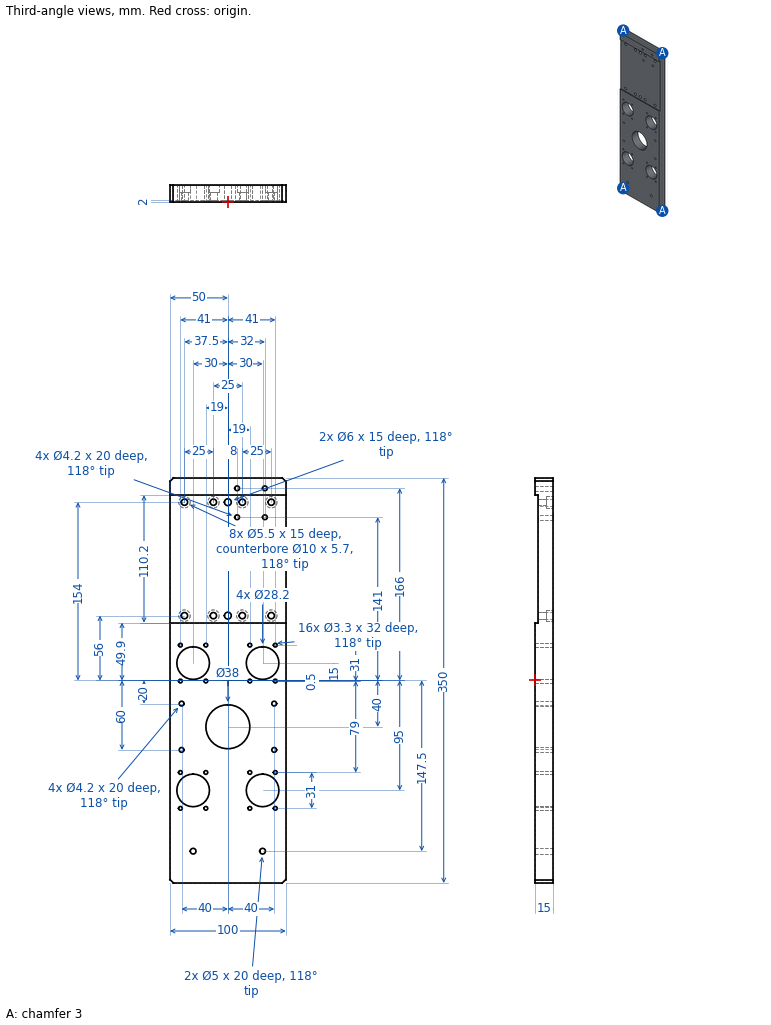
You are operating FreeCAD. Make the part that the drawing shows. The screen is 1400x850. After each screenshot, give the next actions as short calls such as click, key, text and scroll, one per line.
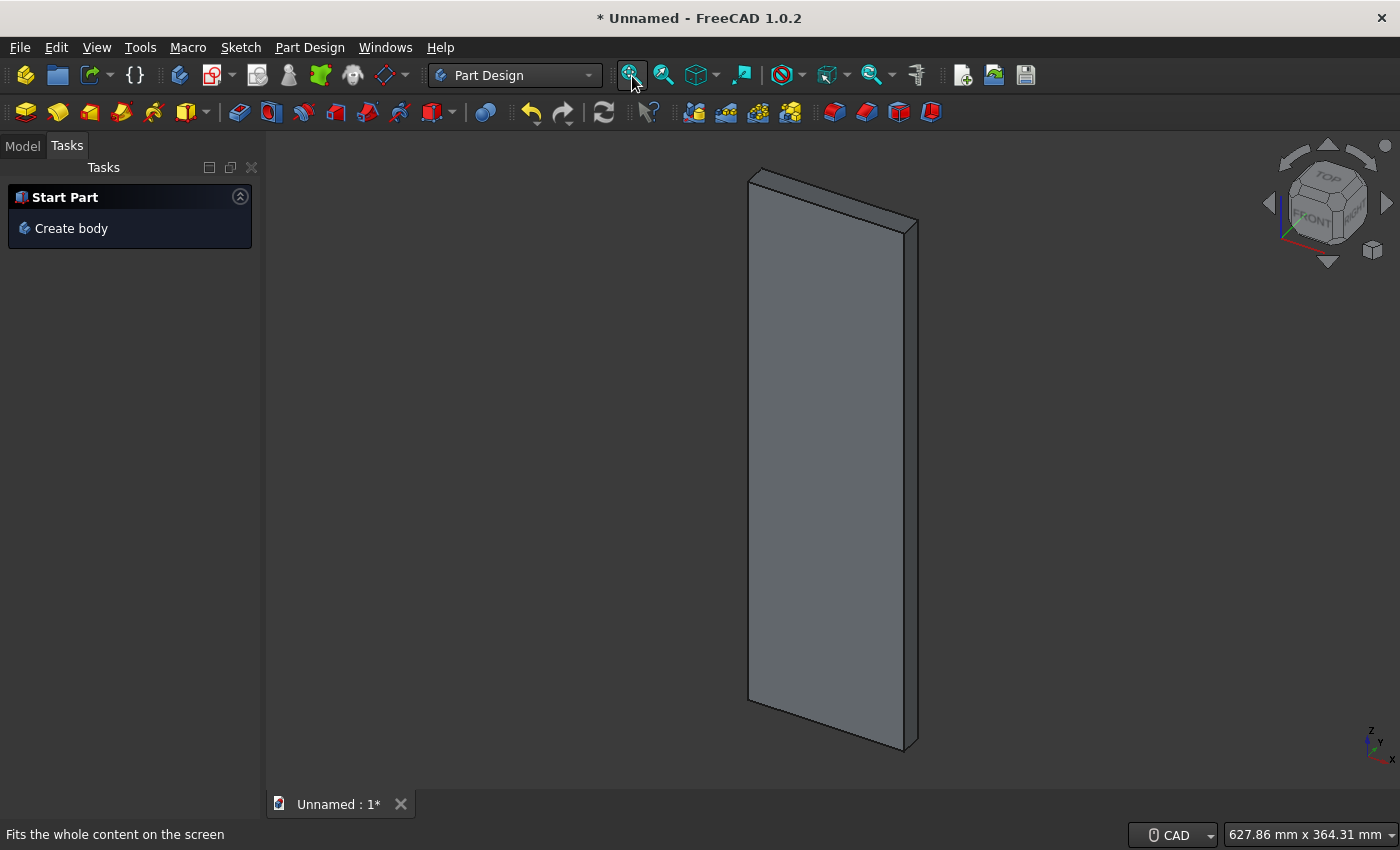
click(826, 318)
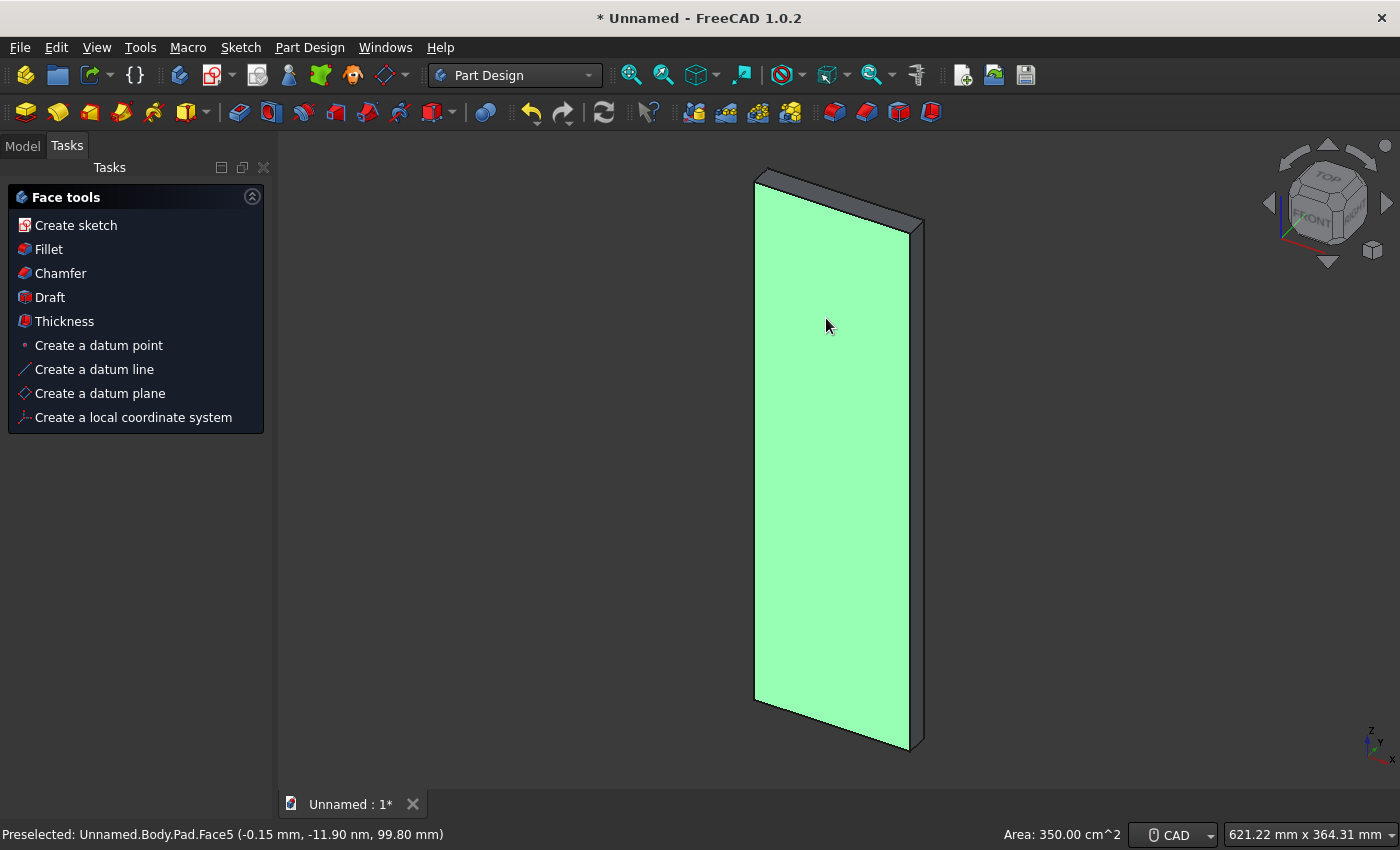
click(212, 76)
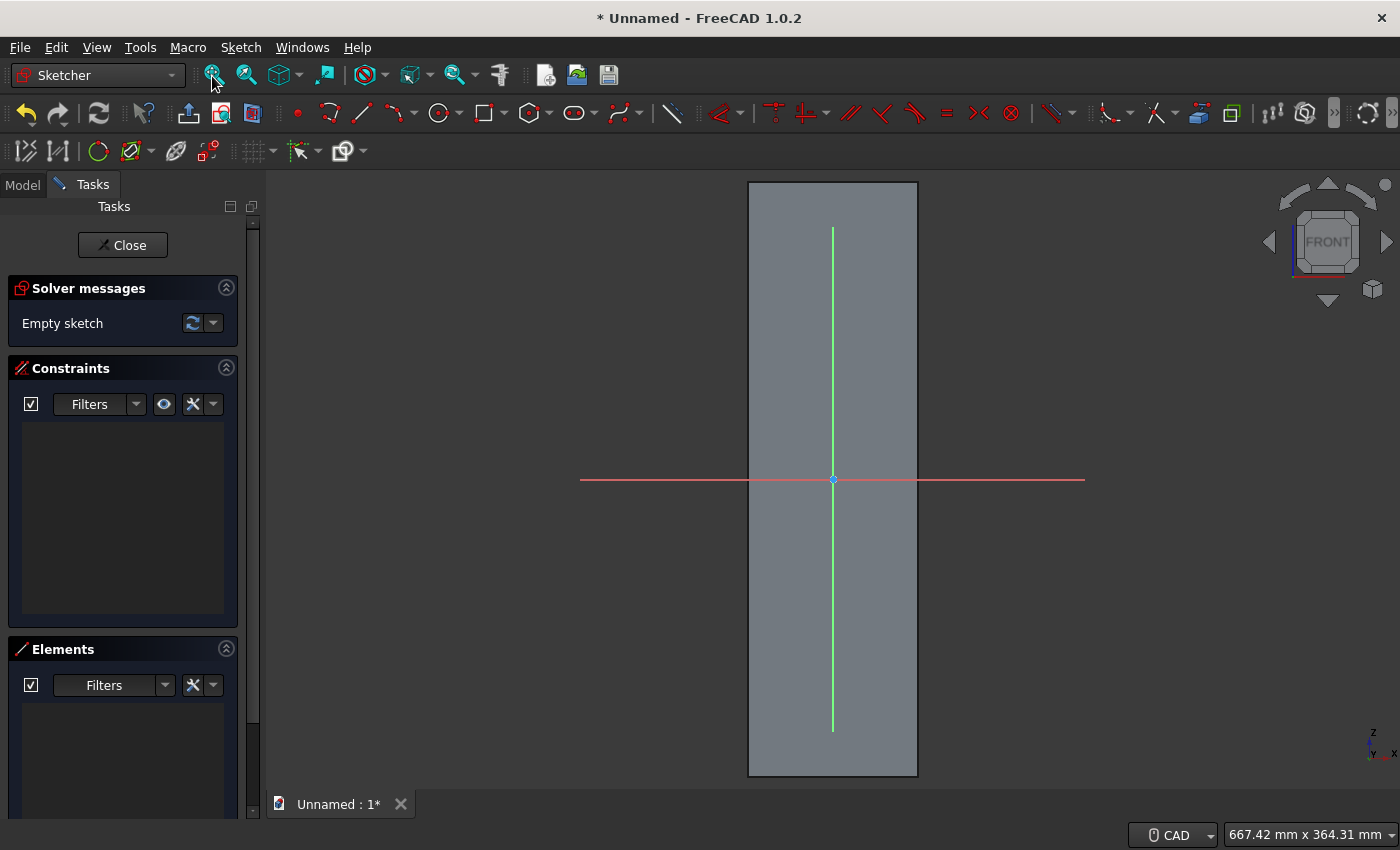
scroll(455, 761, down, 1)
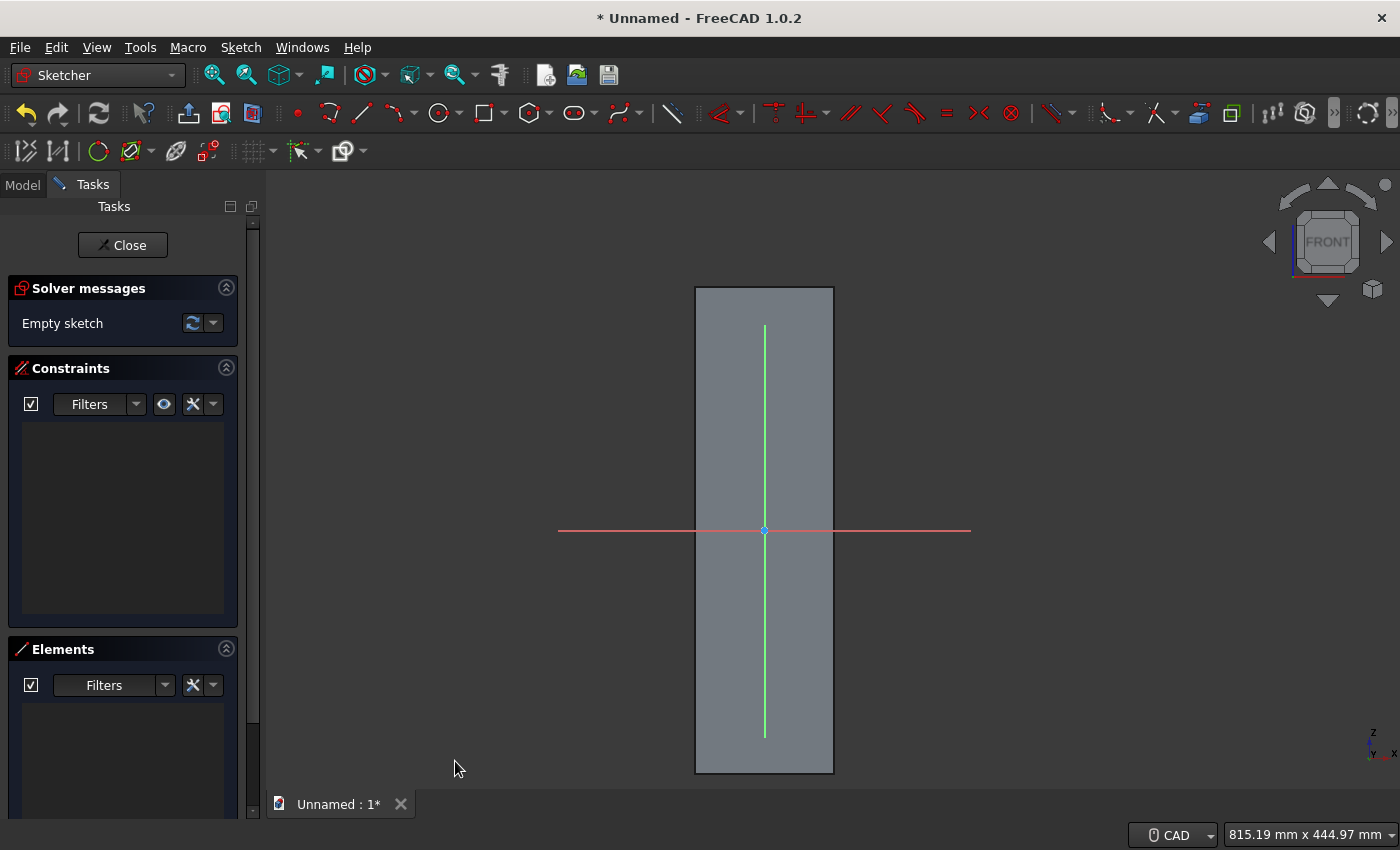
scroll(765, 346, up, 3)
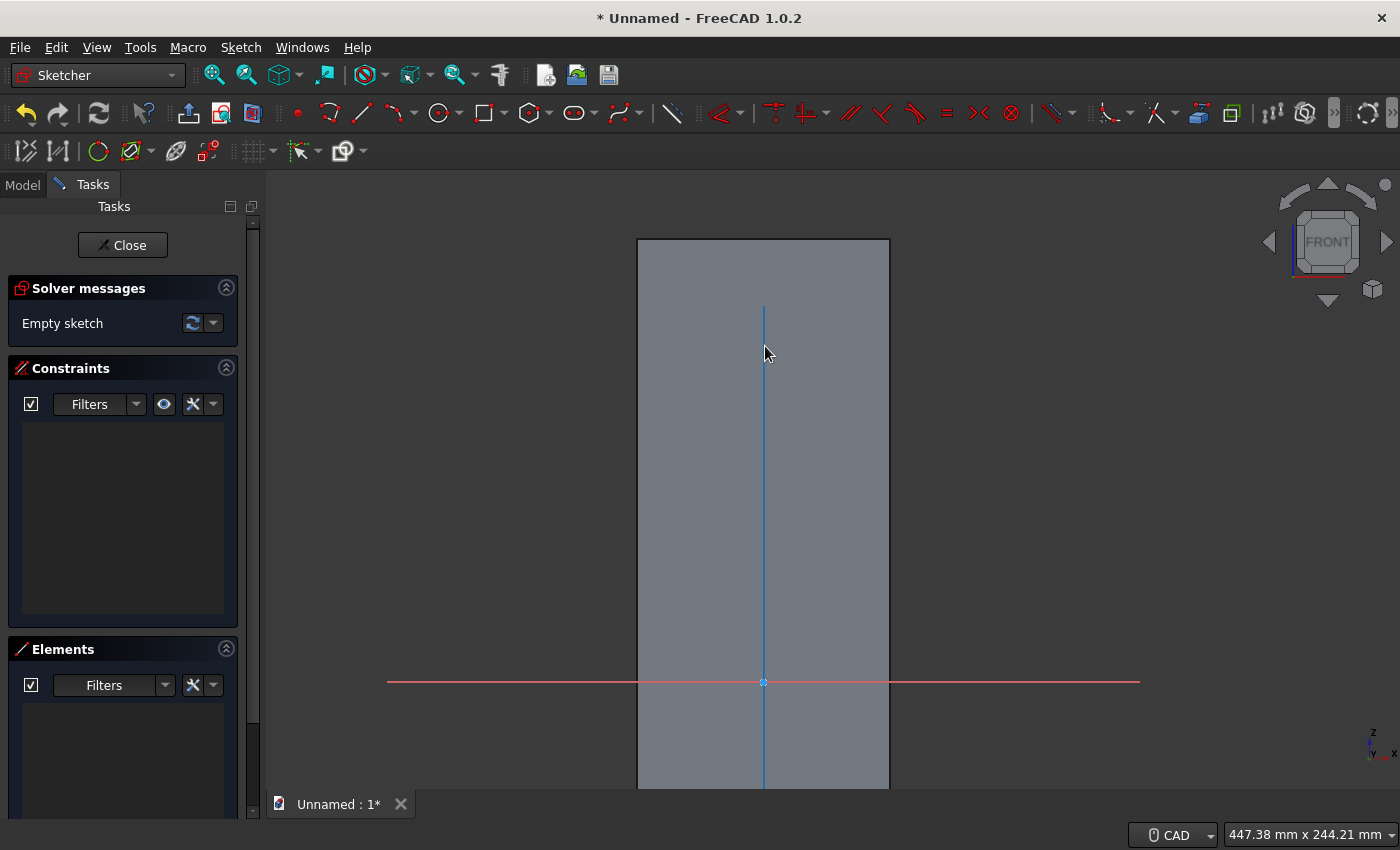
key(g)
key(r)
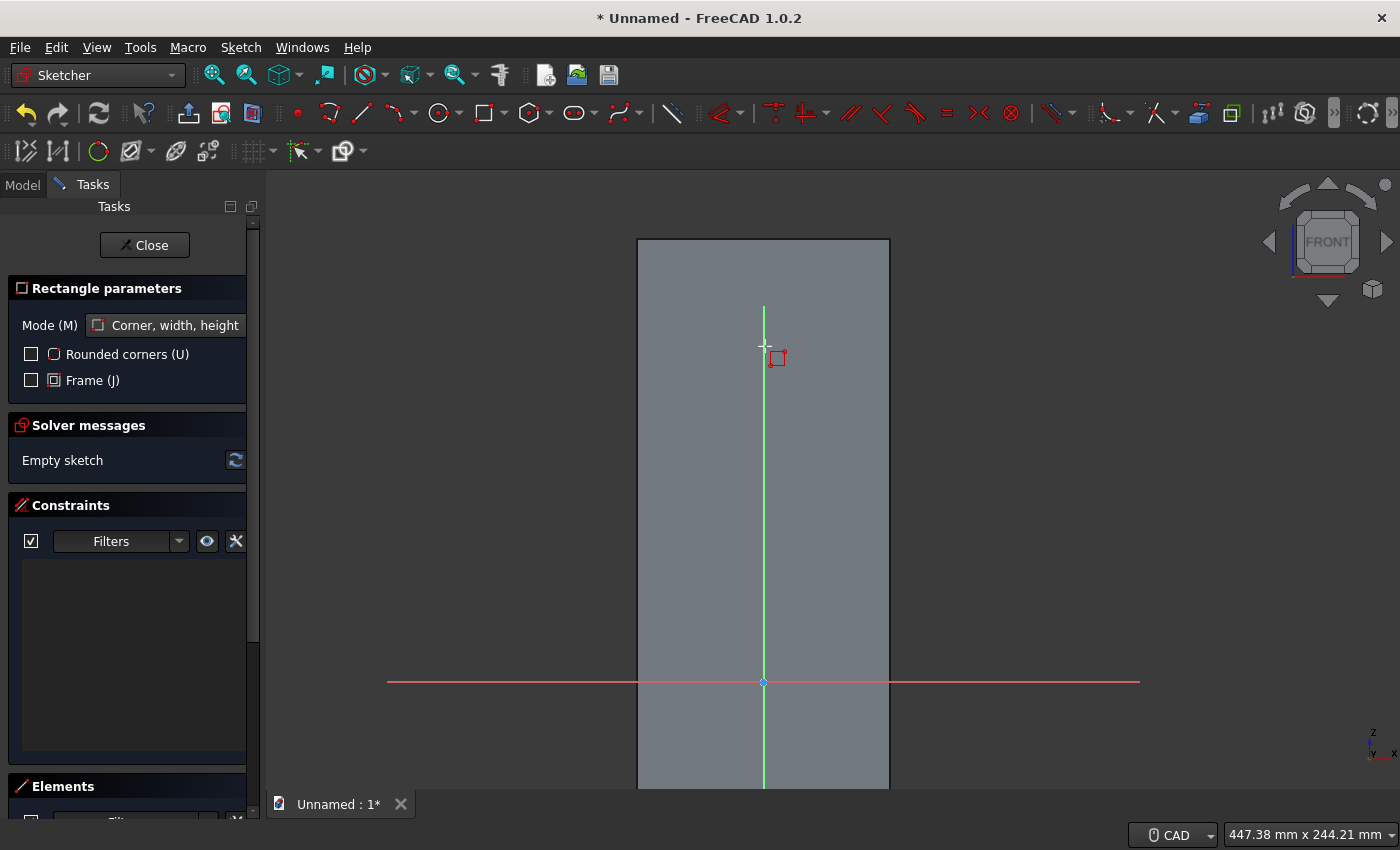
click(637, 277)
click(890, 556)
key(Escape)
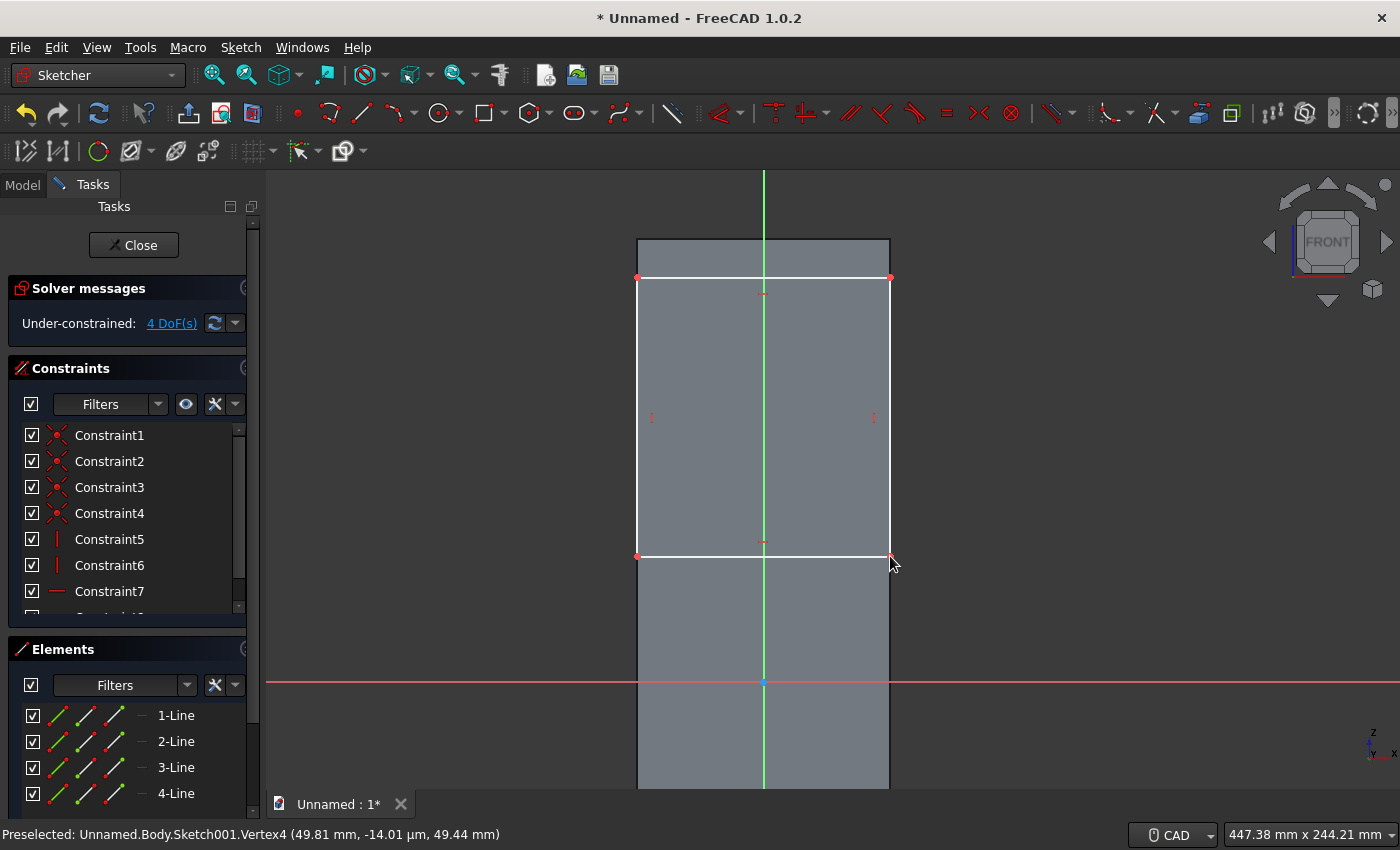
key(d)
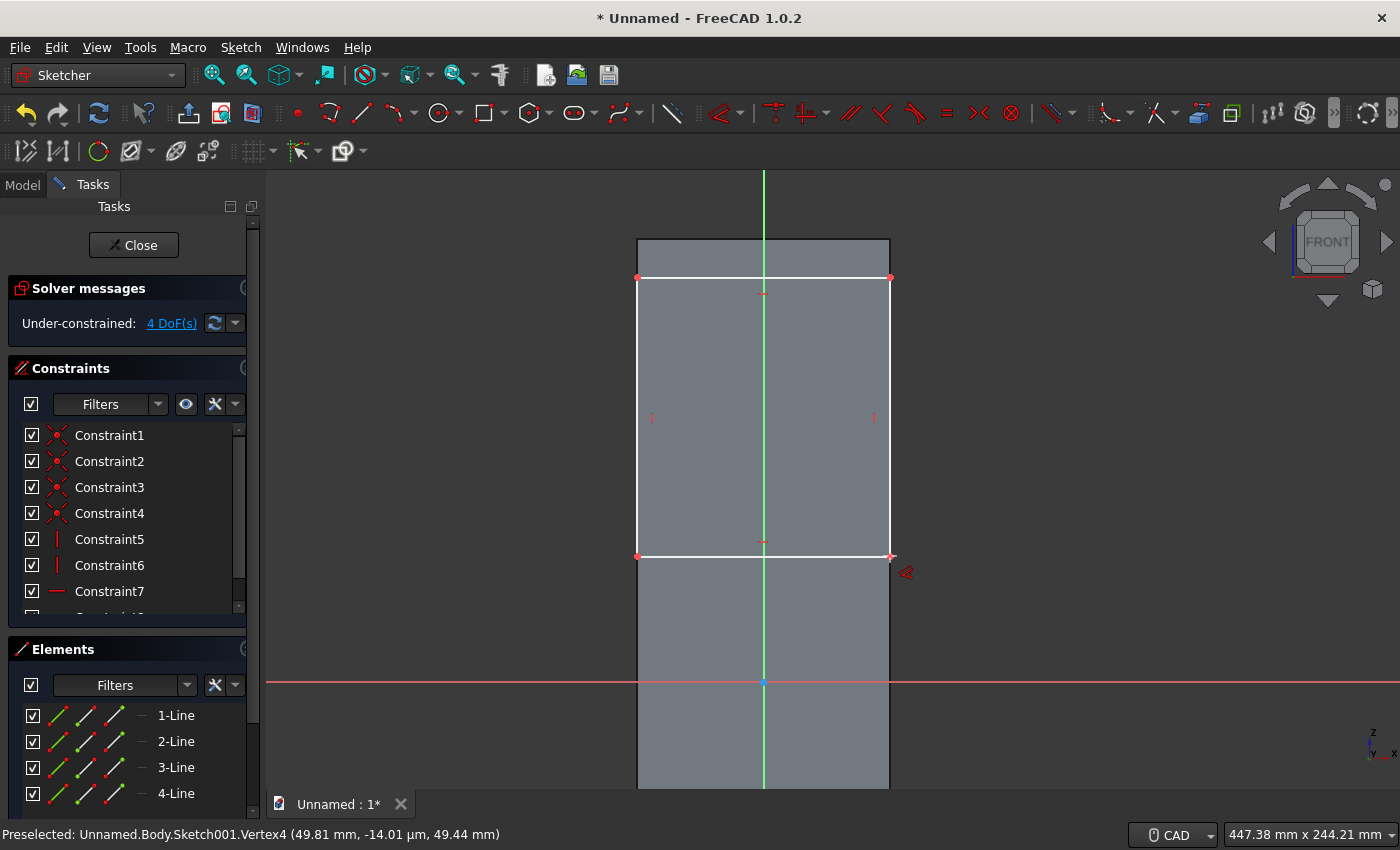
click(713, 557)
click(705, 591)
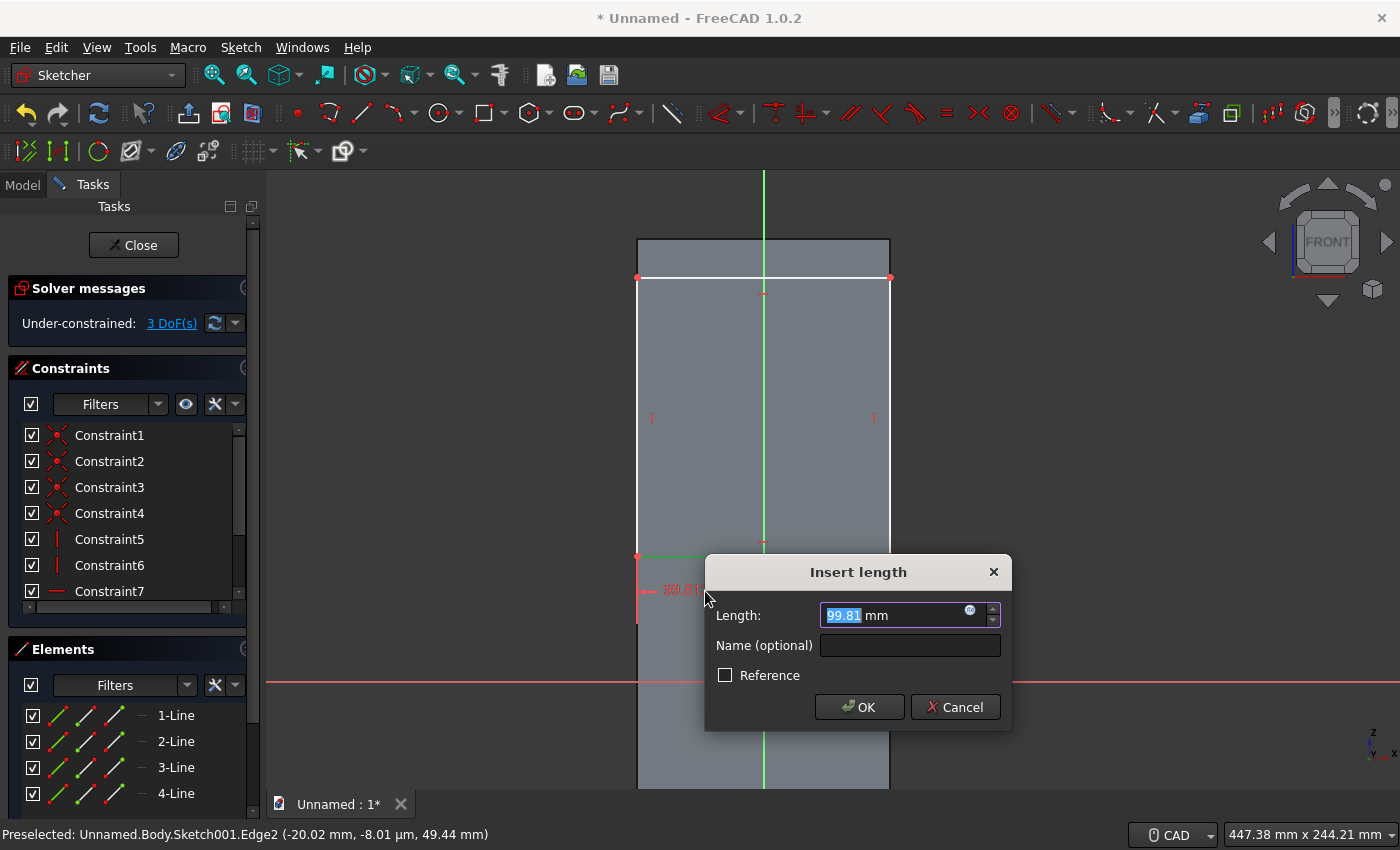
text(100)
key(Return)